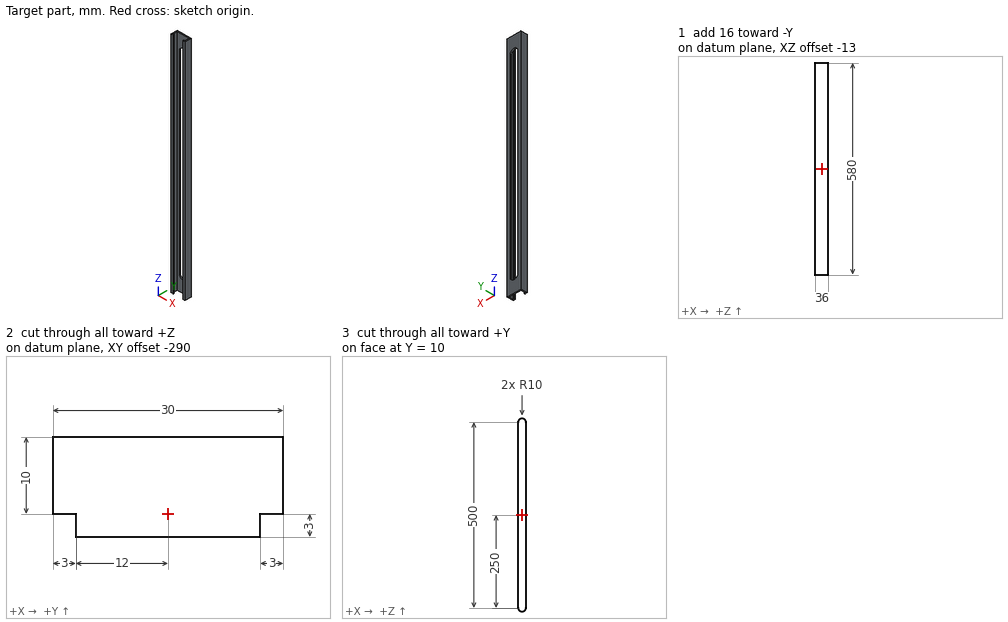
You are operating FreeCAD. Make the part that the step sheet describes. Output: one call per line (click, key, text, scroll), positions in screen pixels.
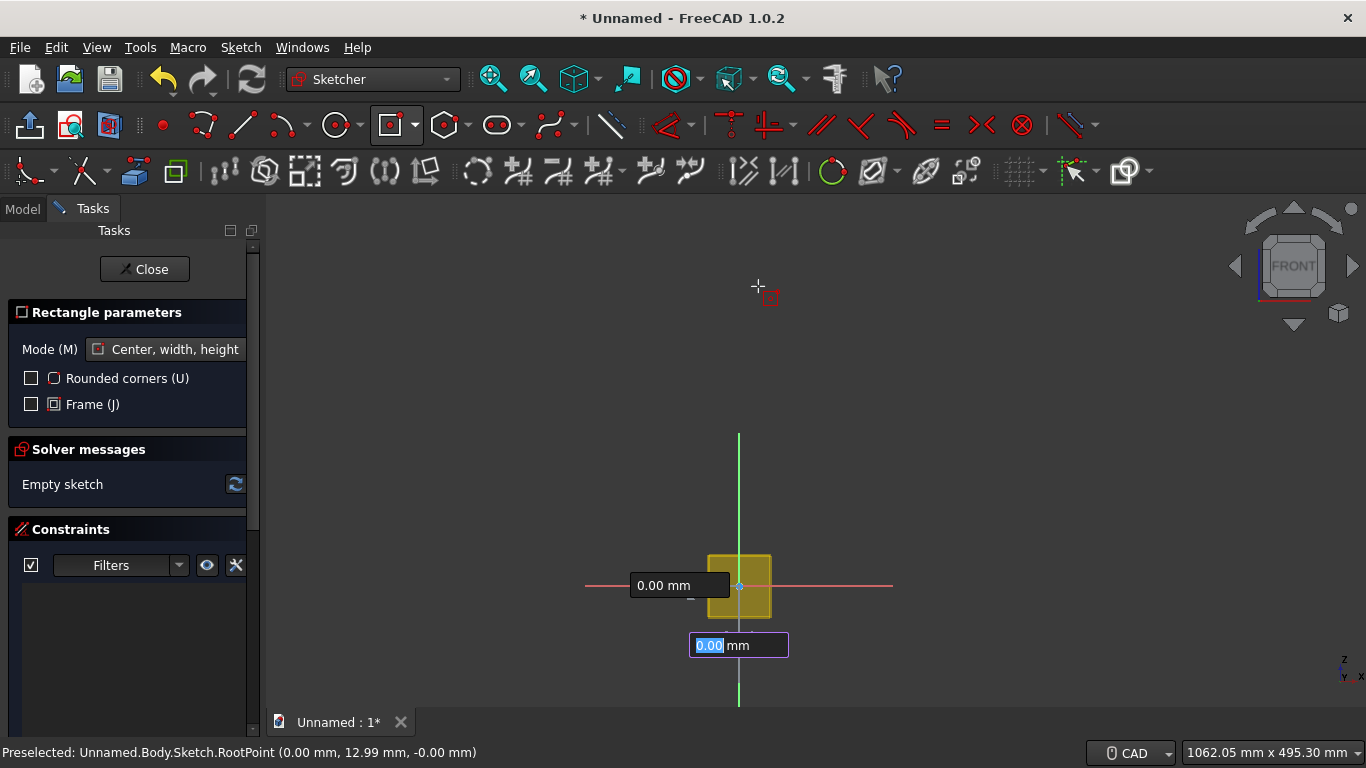
click(758, 286)
key(Escape)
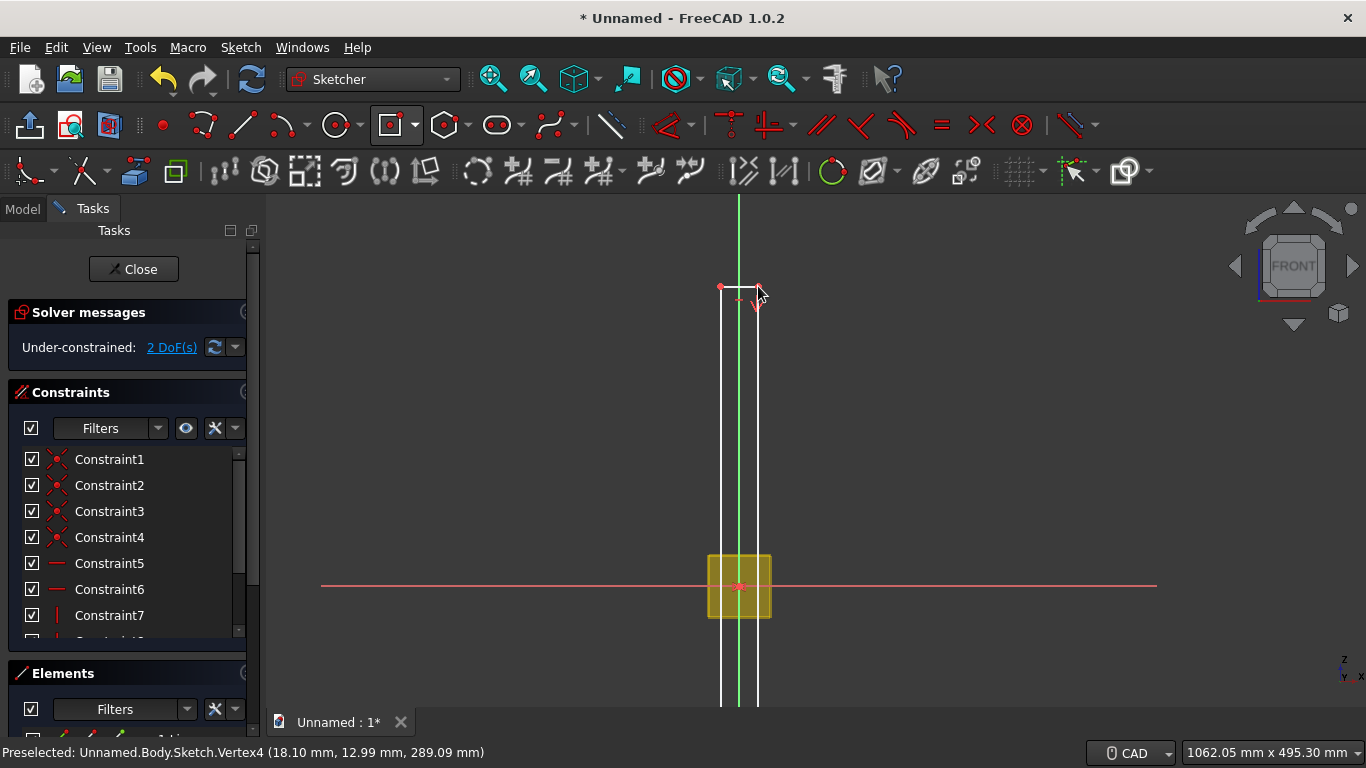
click(666, 126)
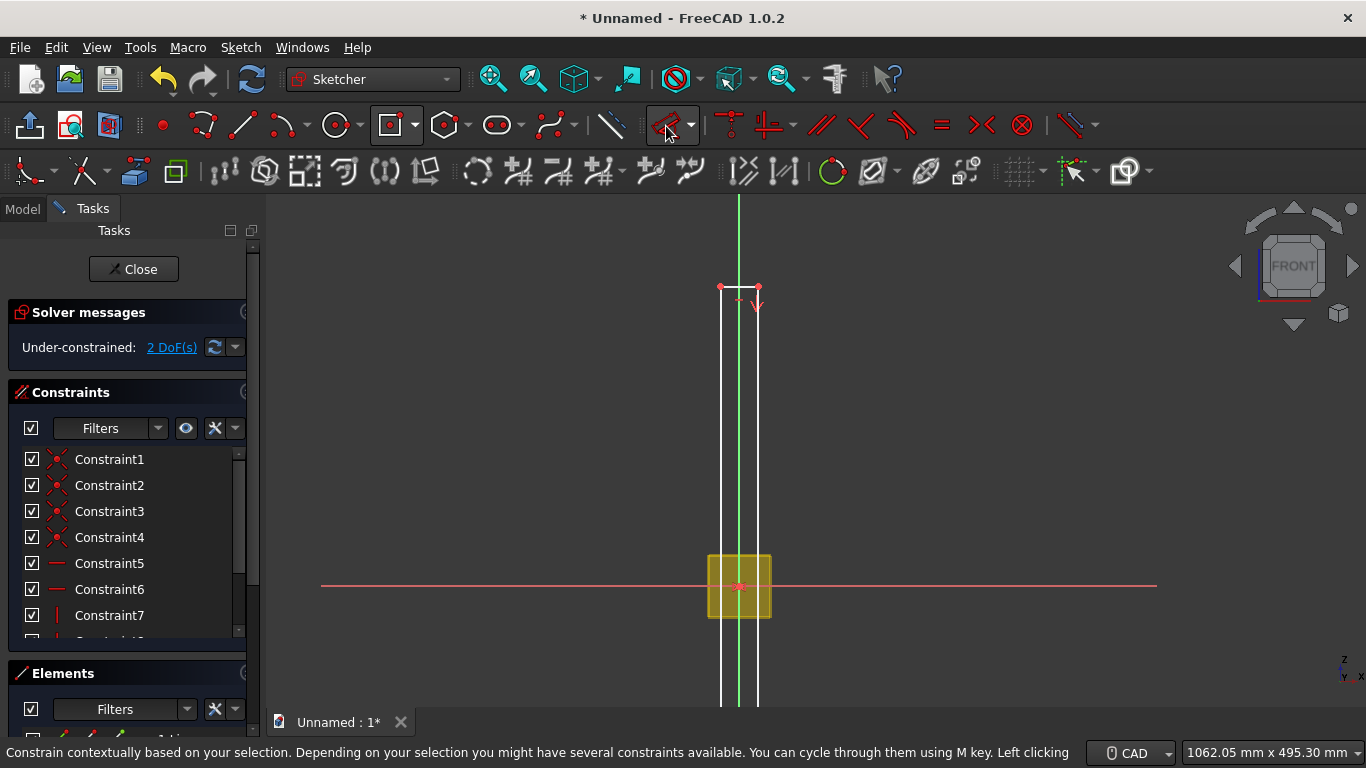
scroll(758, 285, down, 3)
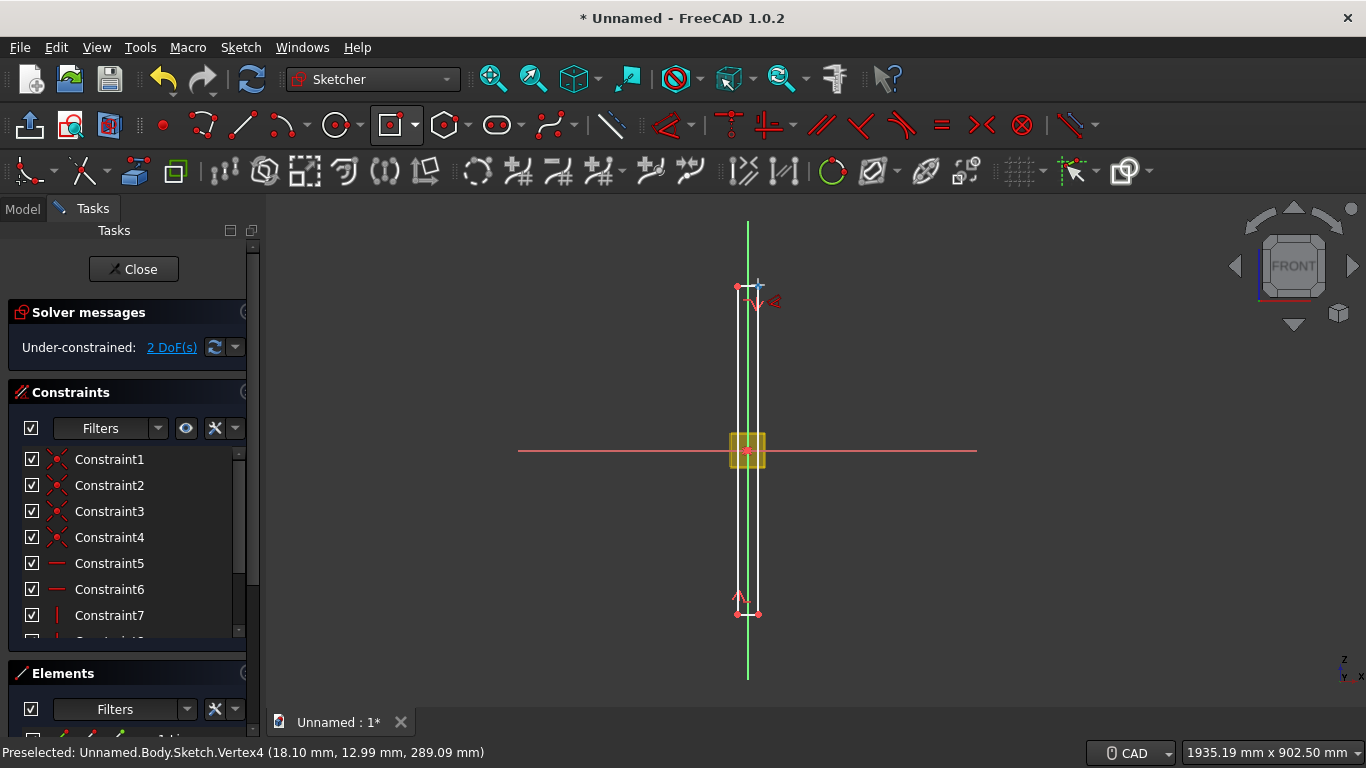
scroll(746, 615, up, 4)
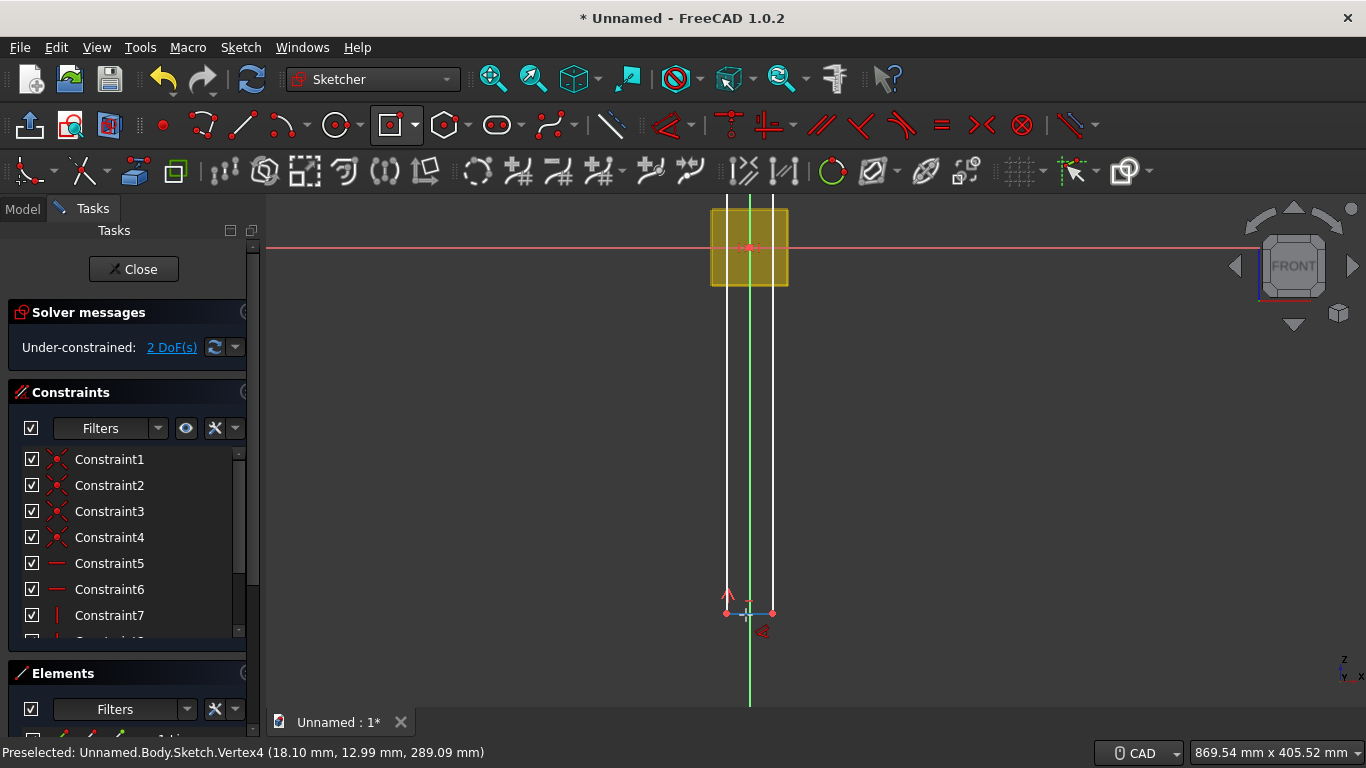
click(745, 614)
click(734, 648)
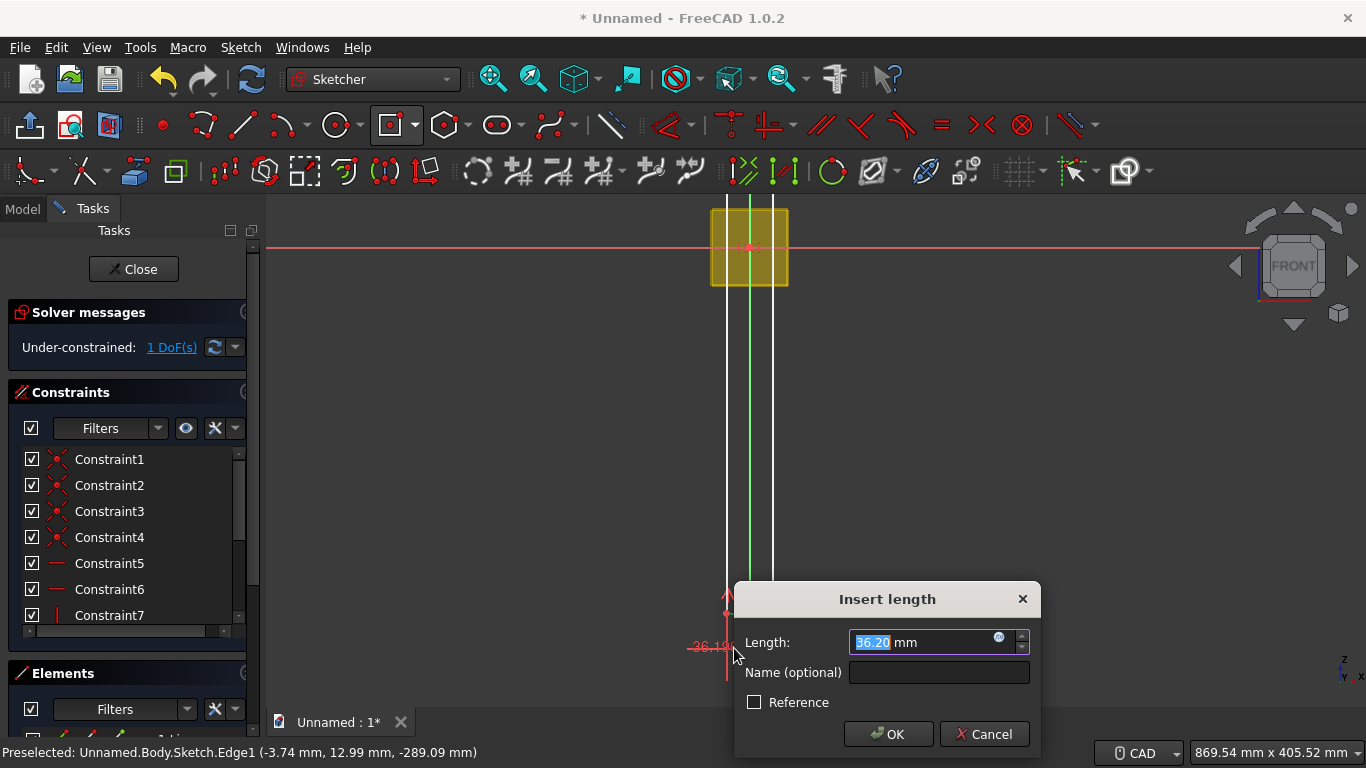
text(36)
key(Return)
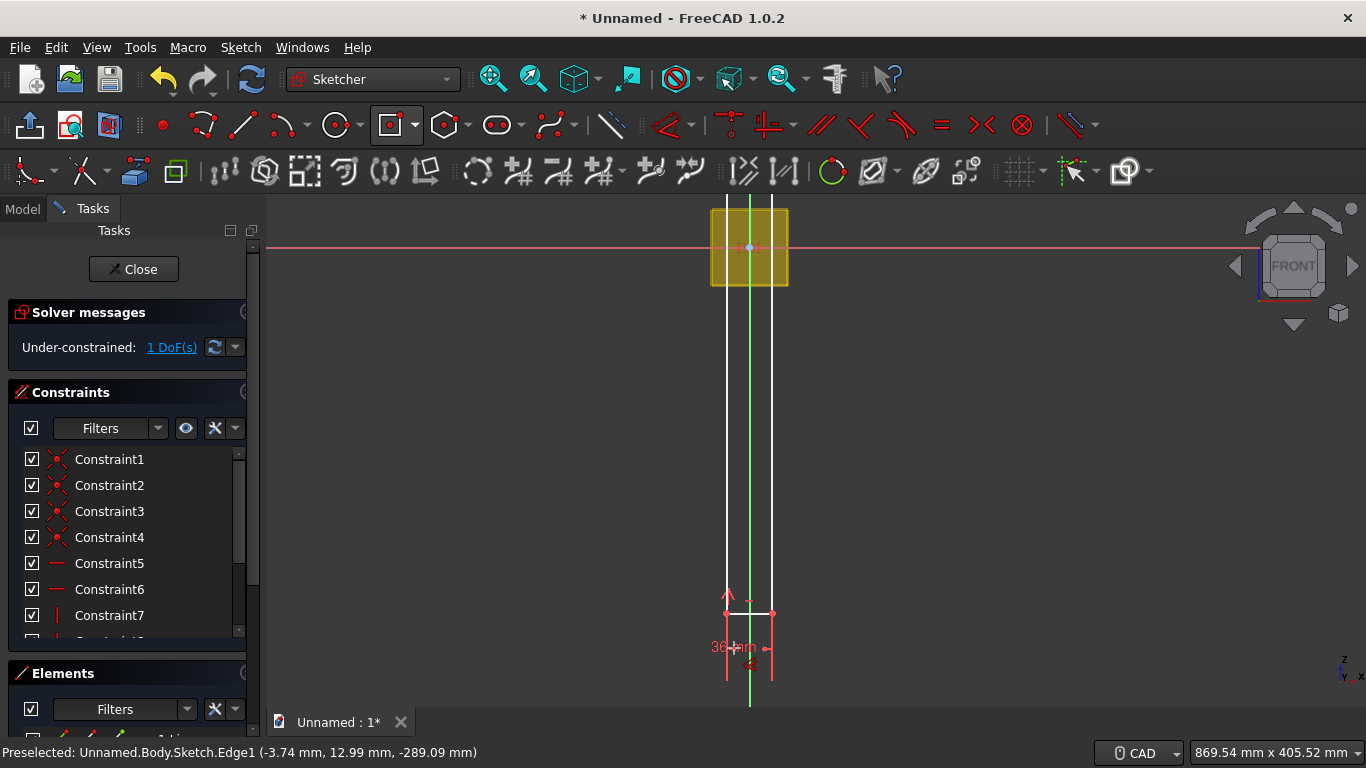
click(772, 394)
click(806, 418)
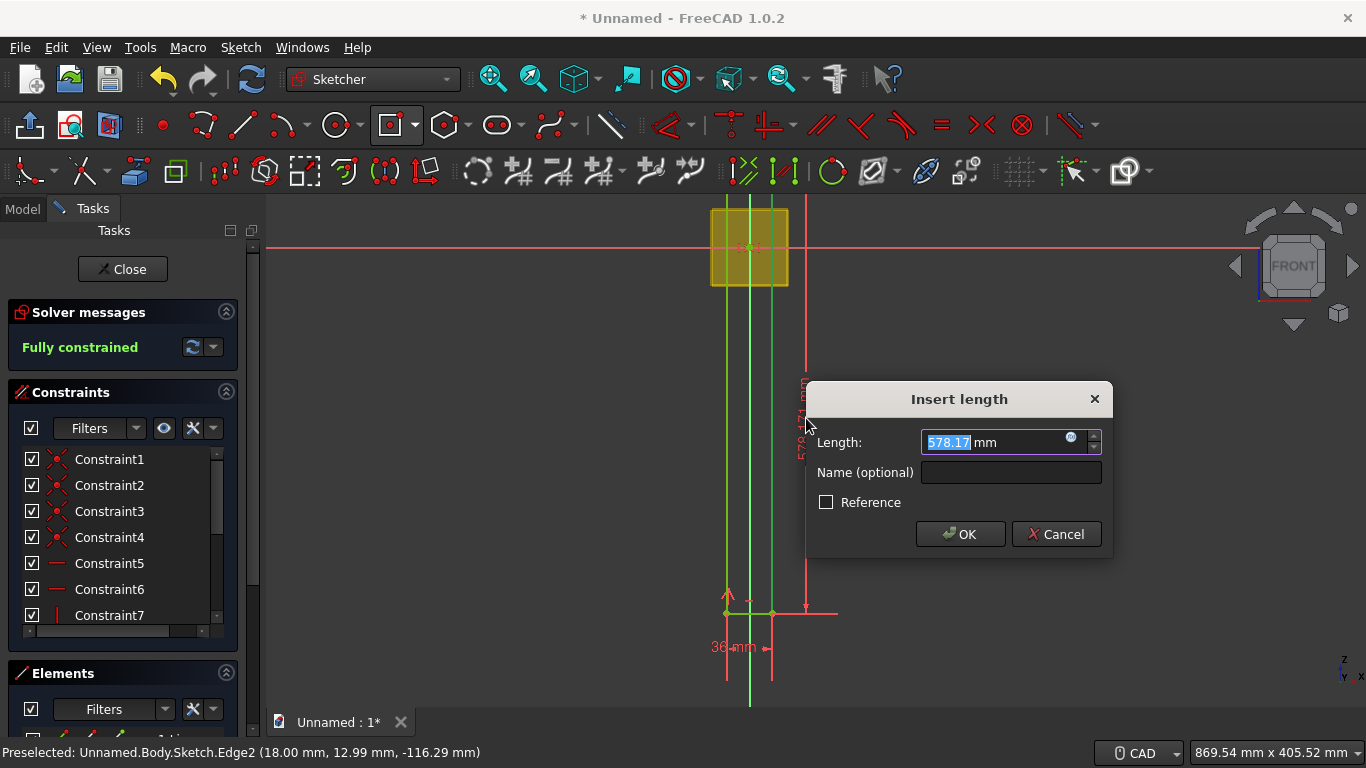
text(580)
key(Return)
key(Escape)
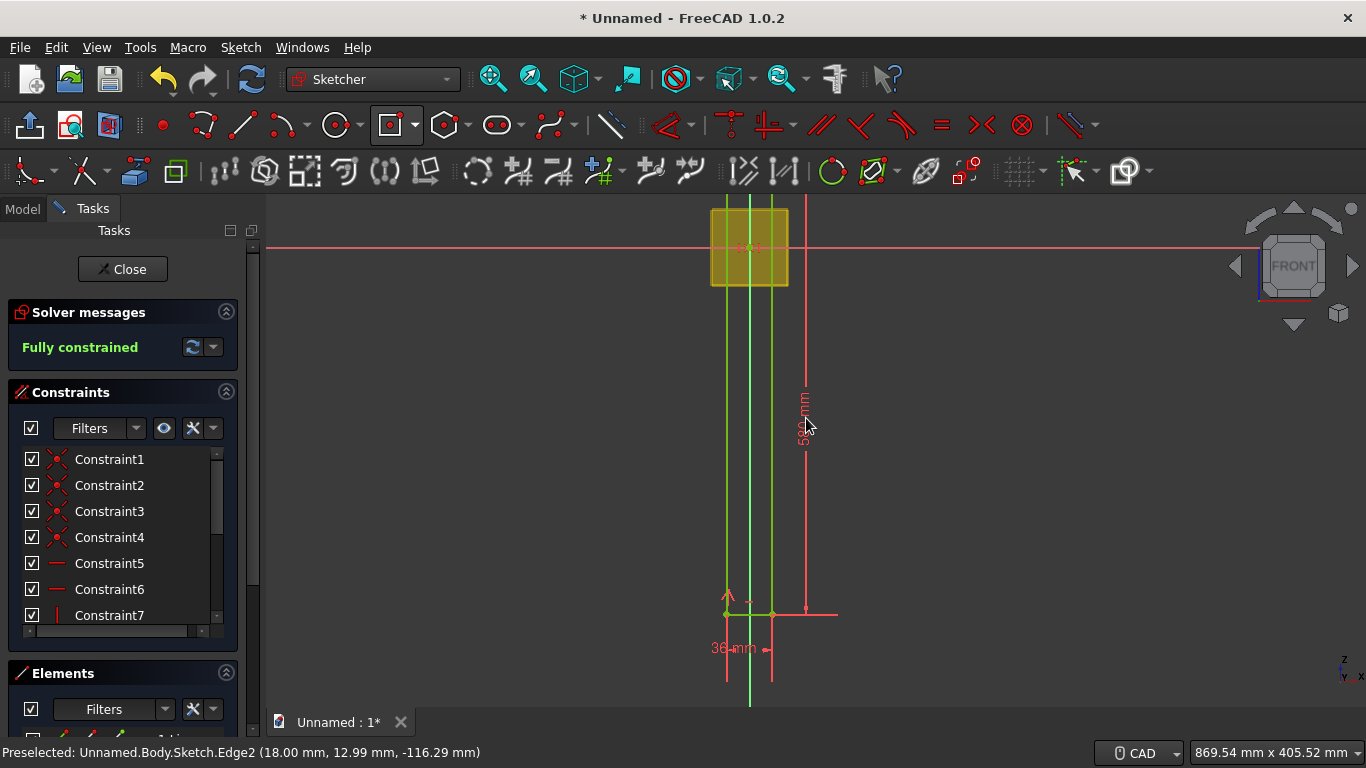
click(123, 269)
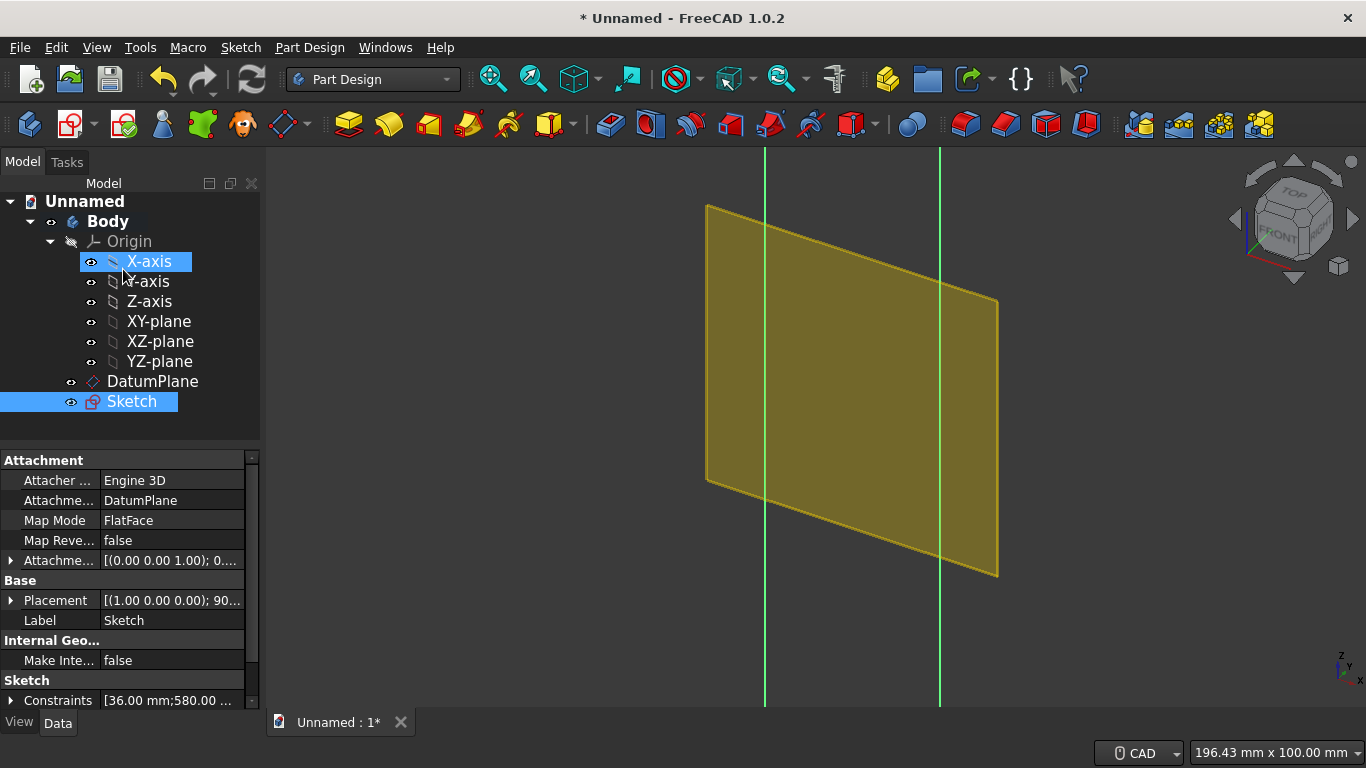
click(350, 124)